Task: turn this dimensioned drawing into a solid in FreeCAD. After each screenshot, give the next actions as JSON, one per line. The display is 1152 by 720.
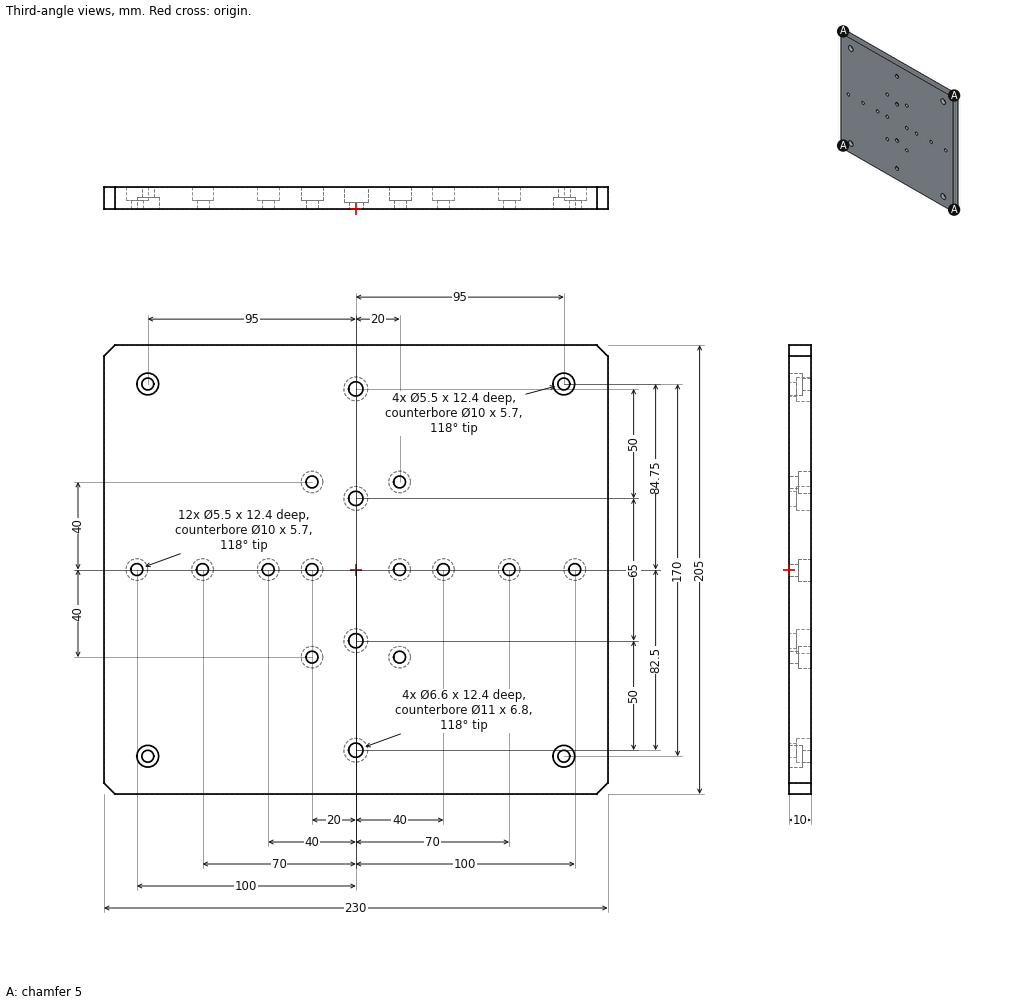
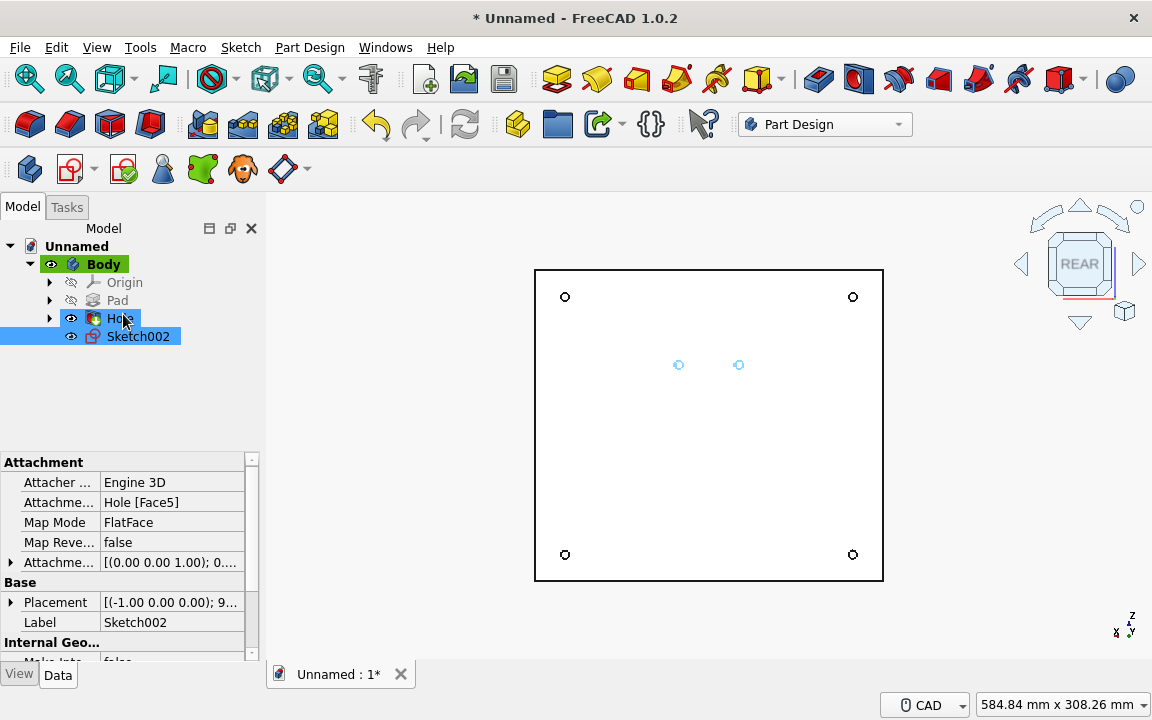
{"action": "left_click", "coordinate": [860, 80]}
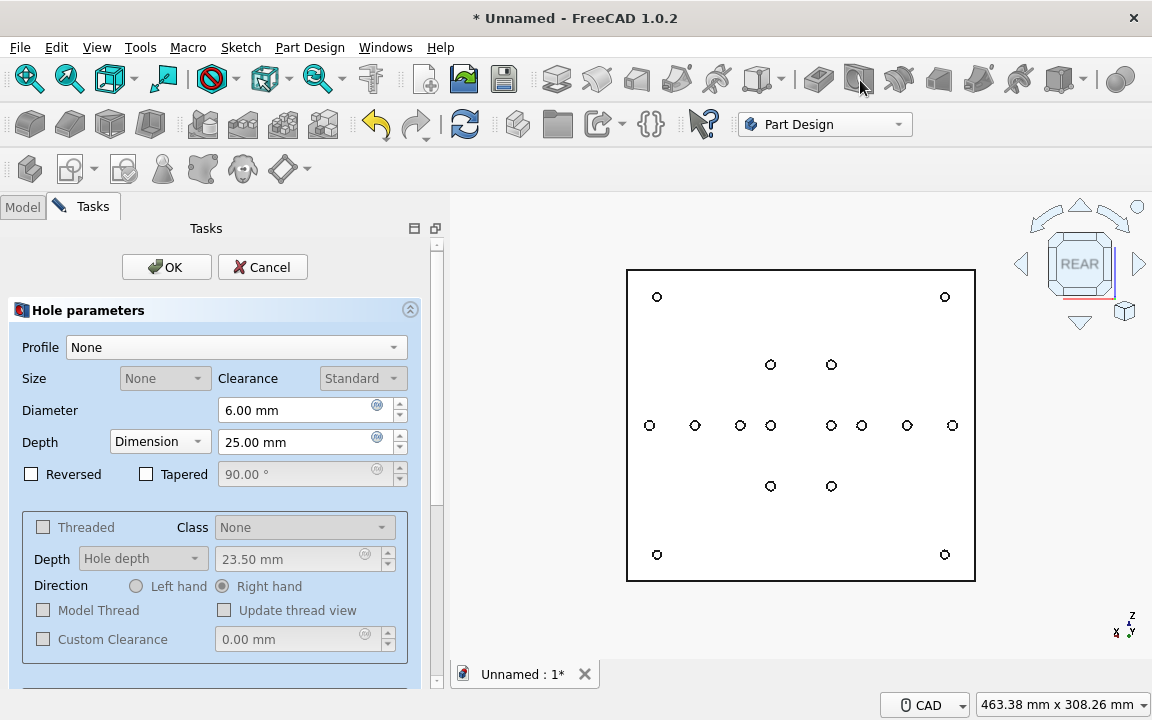
{"action": "triple_click", "coordinate": [305, 410]}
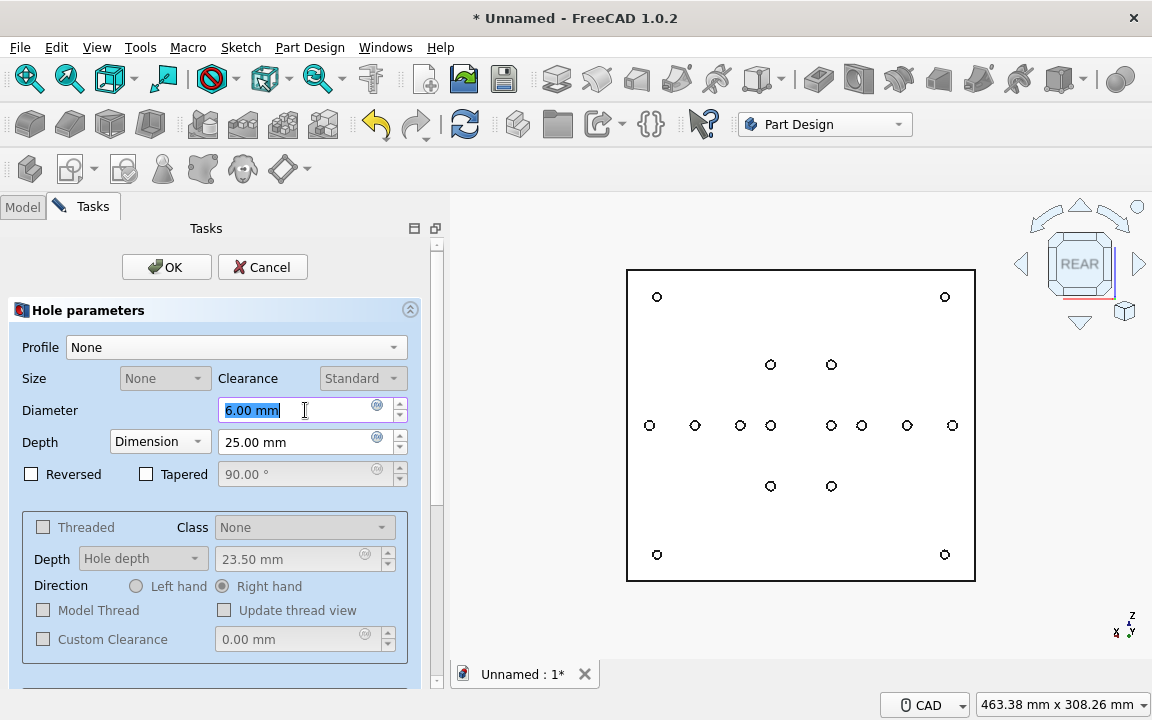
{"action": "type", "text": "5.5"}
{"action": "key", "text": "Tab"}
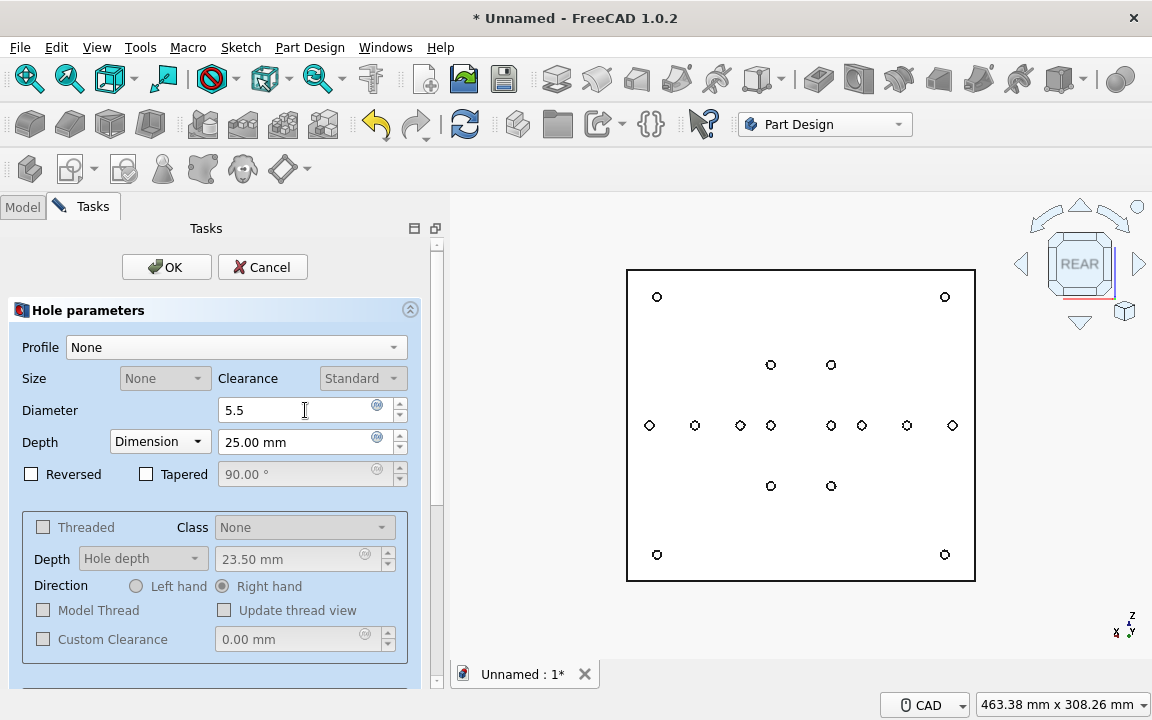
{"action": "triple_click", "coordinate": [305, 442]}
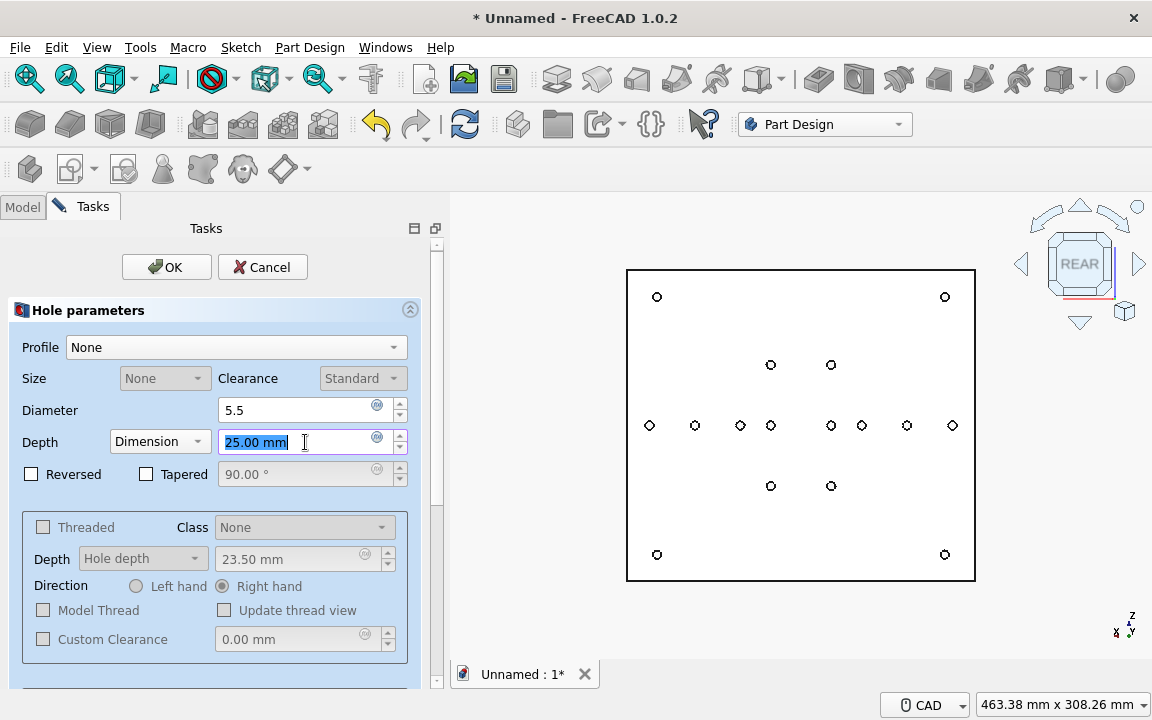
{"action": "type", "text": "12.4"}
{"action": "key", "text": "Tab"}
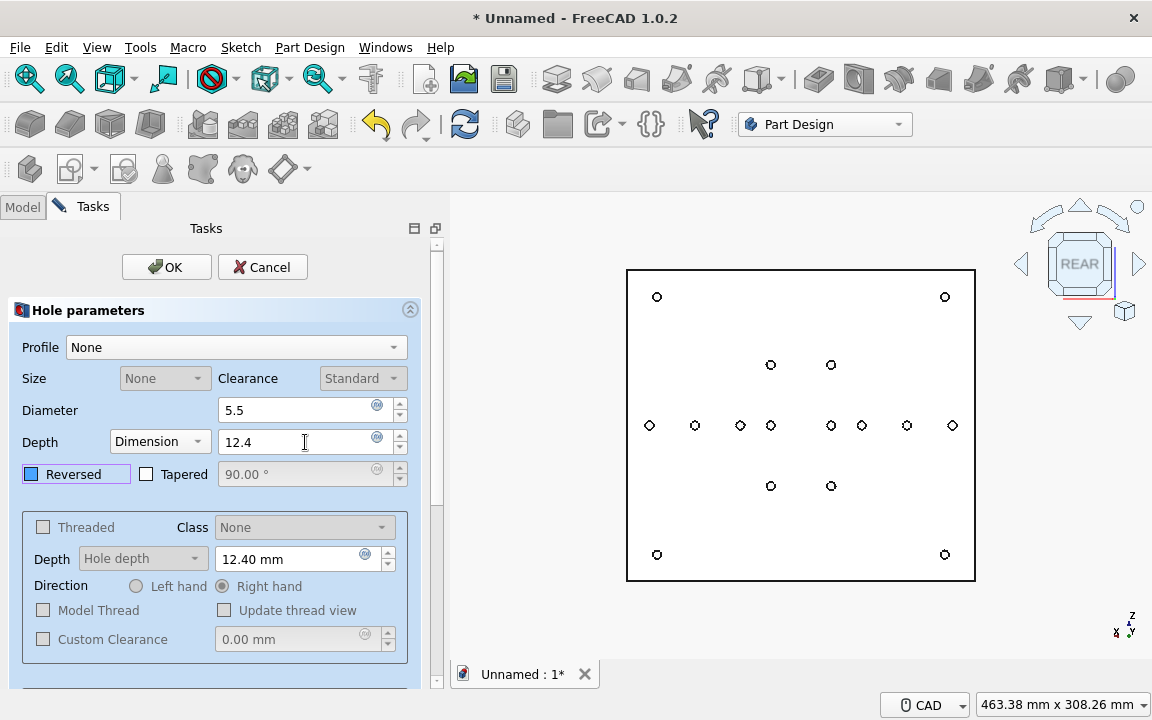
{"action": "scroll", "coordinate": [437, 463], "scroll_direction": "down", "scroll_amount": 2}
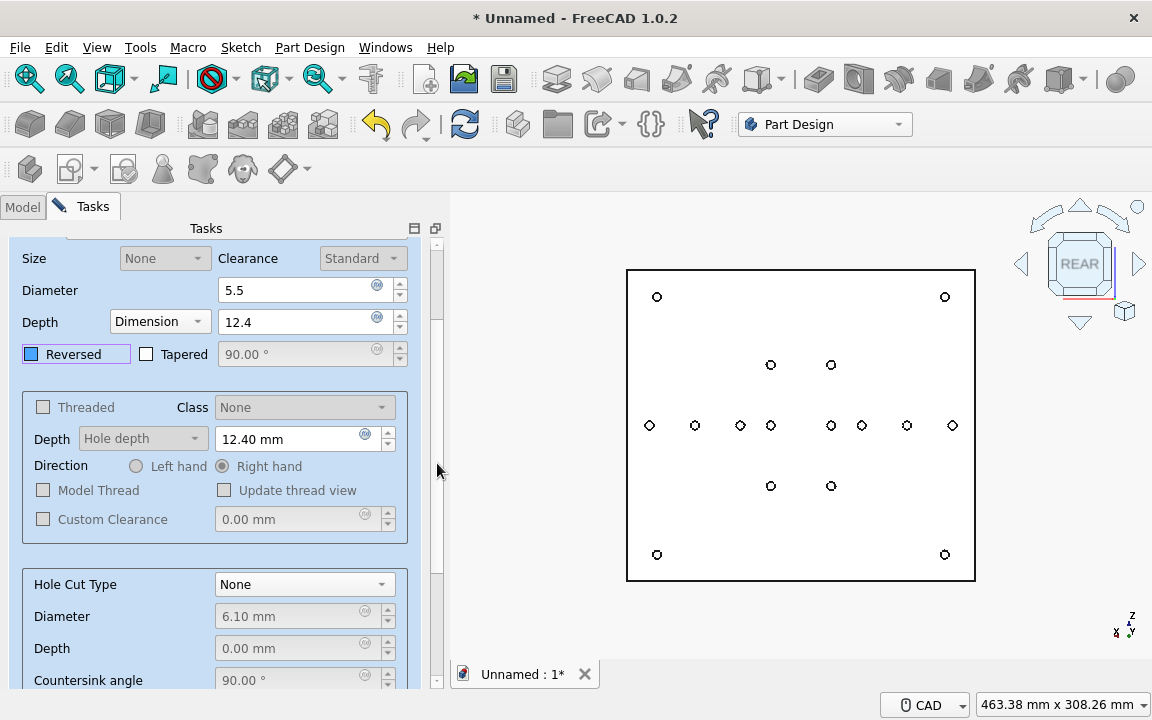
{"action": "left_click", "coordinate": [306, 584]}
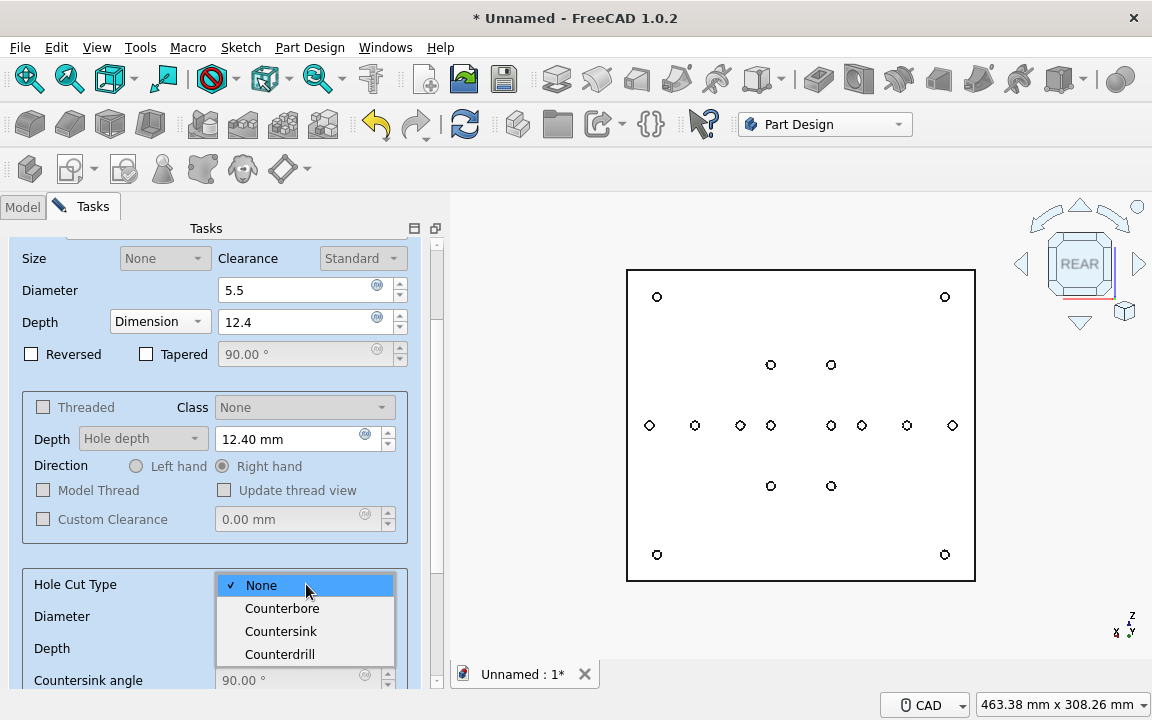
{"action": "left_click", "coordinate": [304, 608]}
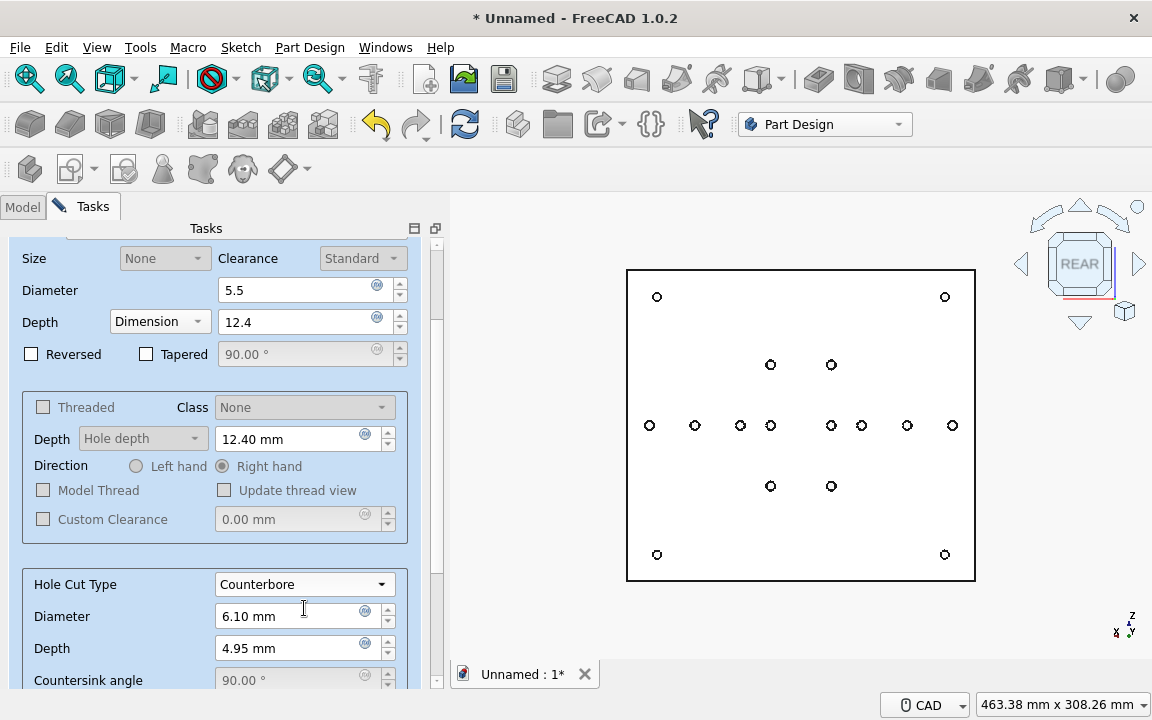
{"action": "triple_click", "coordinate": [298, 616]}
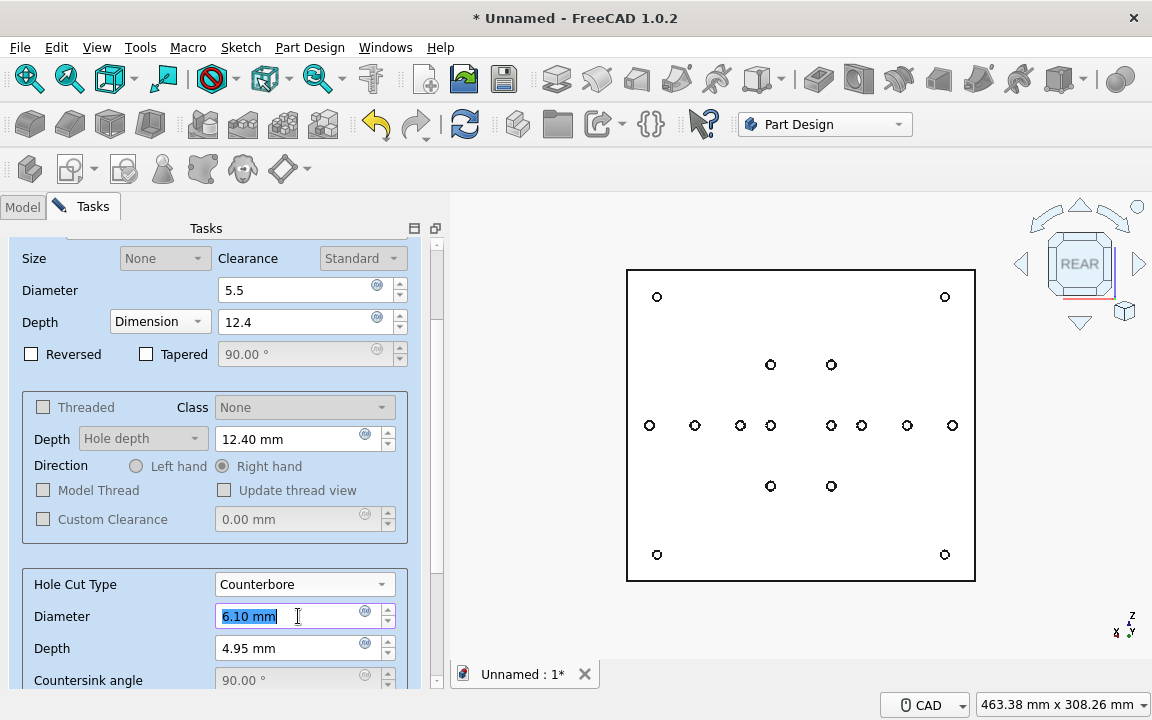
{"action": "type", "text": "10"}
{"action": "key", "text": "Tab"}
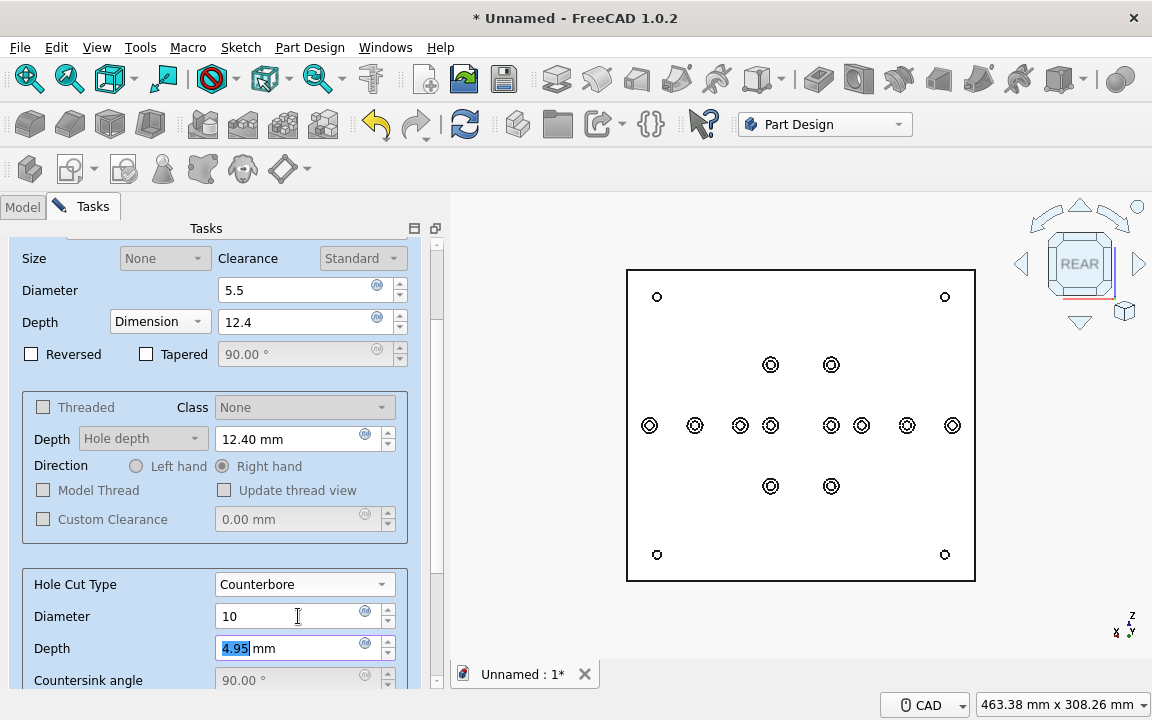
{"action": "type", "text": "5.7"}
{"action": "key", "text": "Tab"}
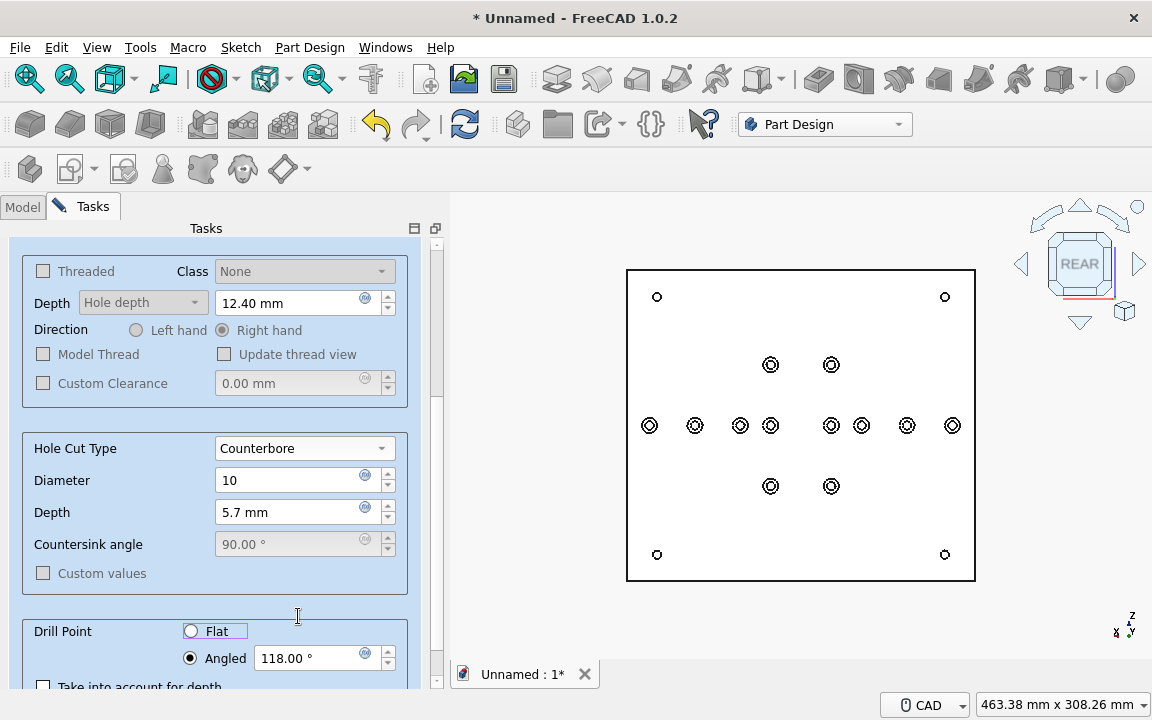
{"action": "scroll", "coordinate": [437, 463], "scroll_direction": "up", "scroll_amount": 6}